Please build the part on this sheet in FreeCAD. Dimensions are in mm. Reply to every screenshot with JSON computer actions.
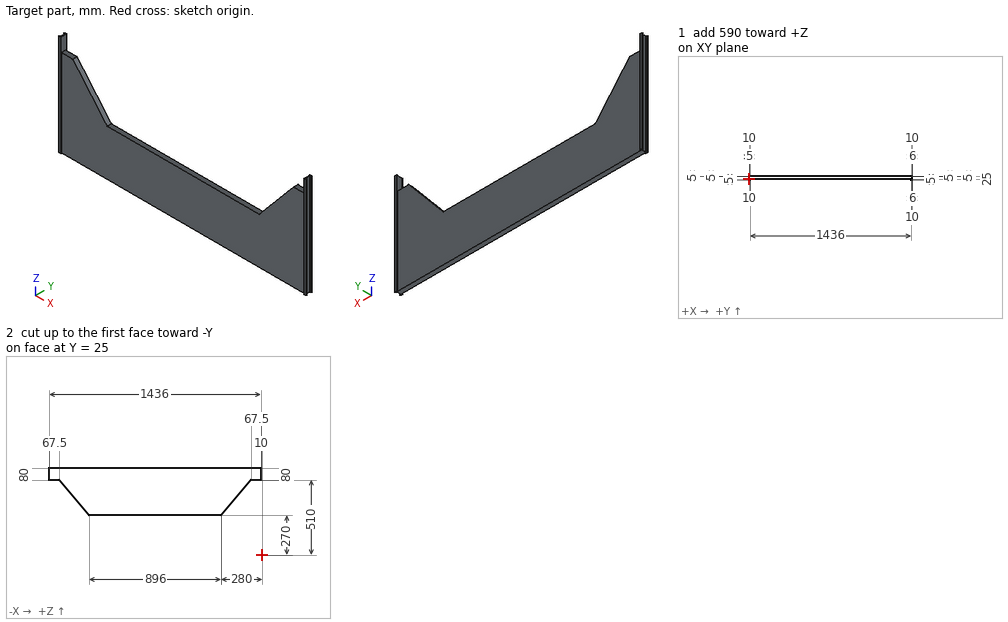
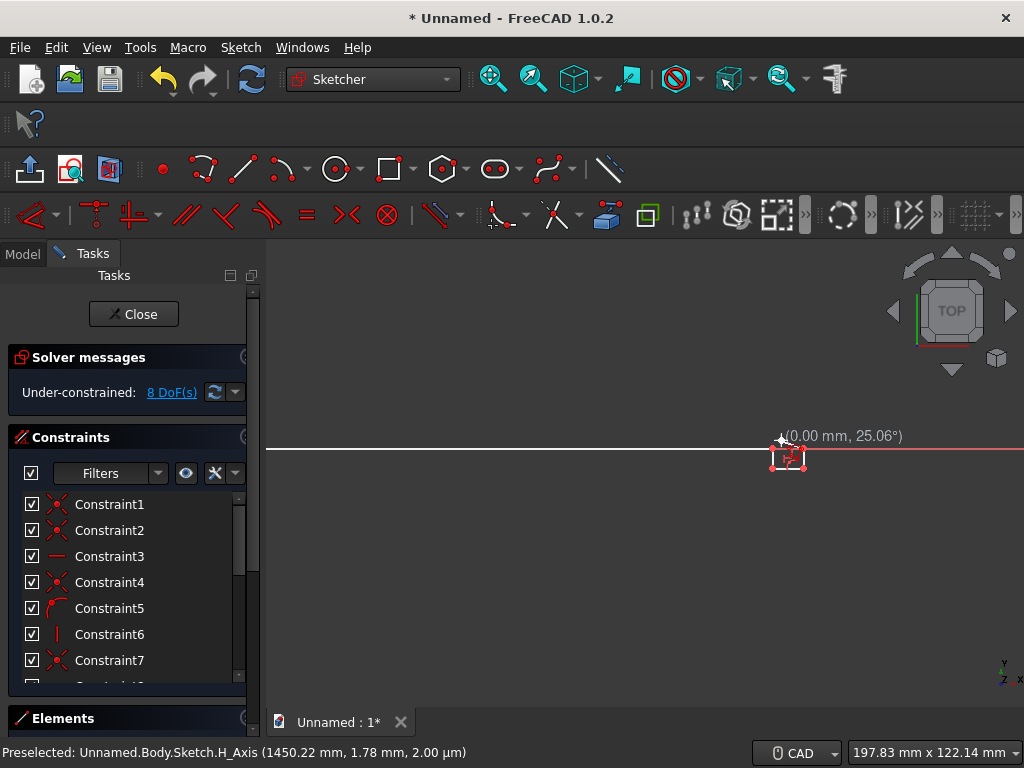
{"action": "scroll", "coordinate": [782, 479], "scroll_direction": "down", "scroll_amount": 13}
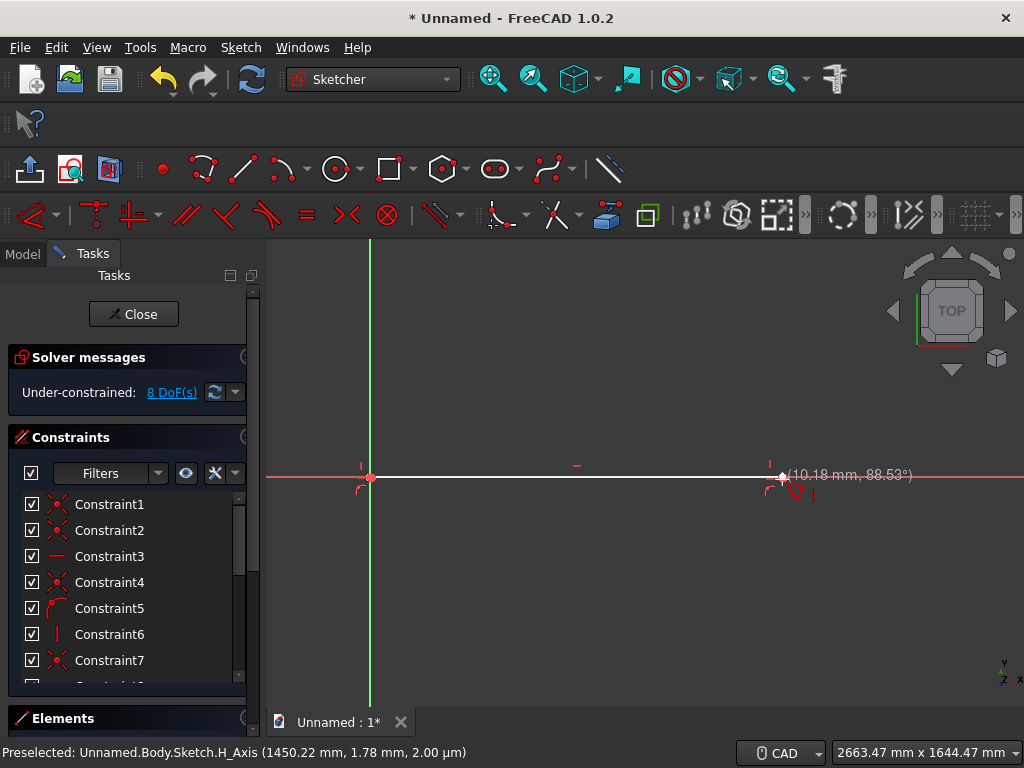
{"action": "scroll", "coordinate": [783, 470], "scroll_direction": "up", "scroll_amount": 5}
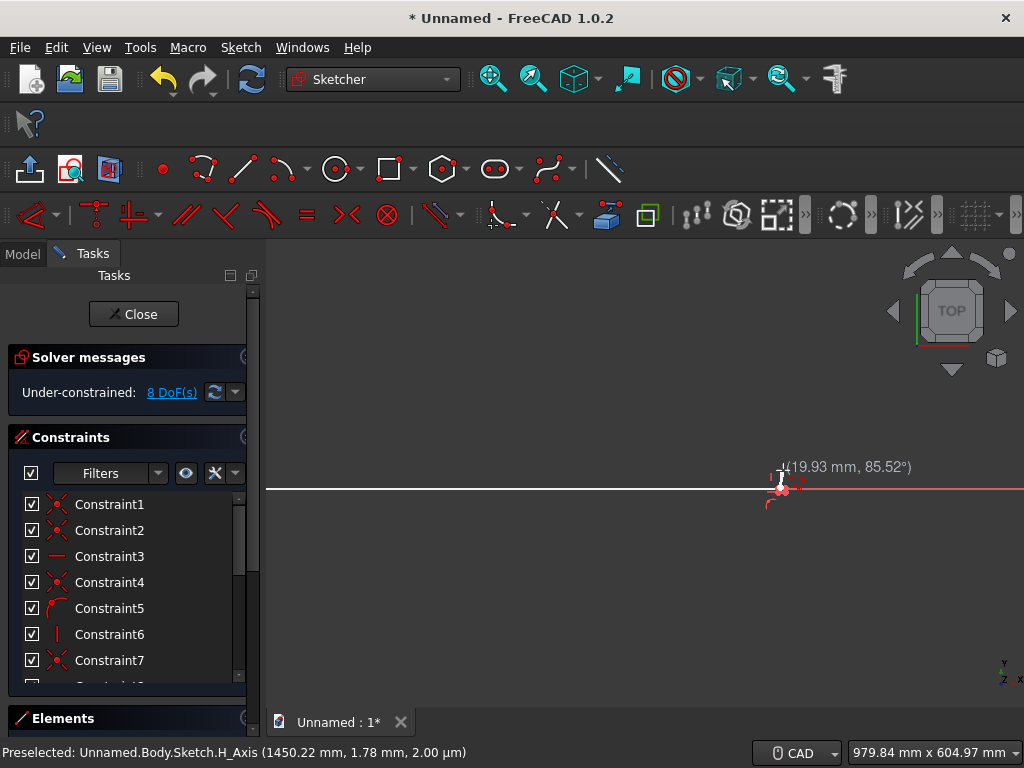
{"action": "left_click", "coordinate": [781, 469]}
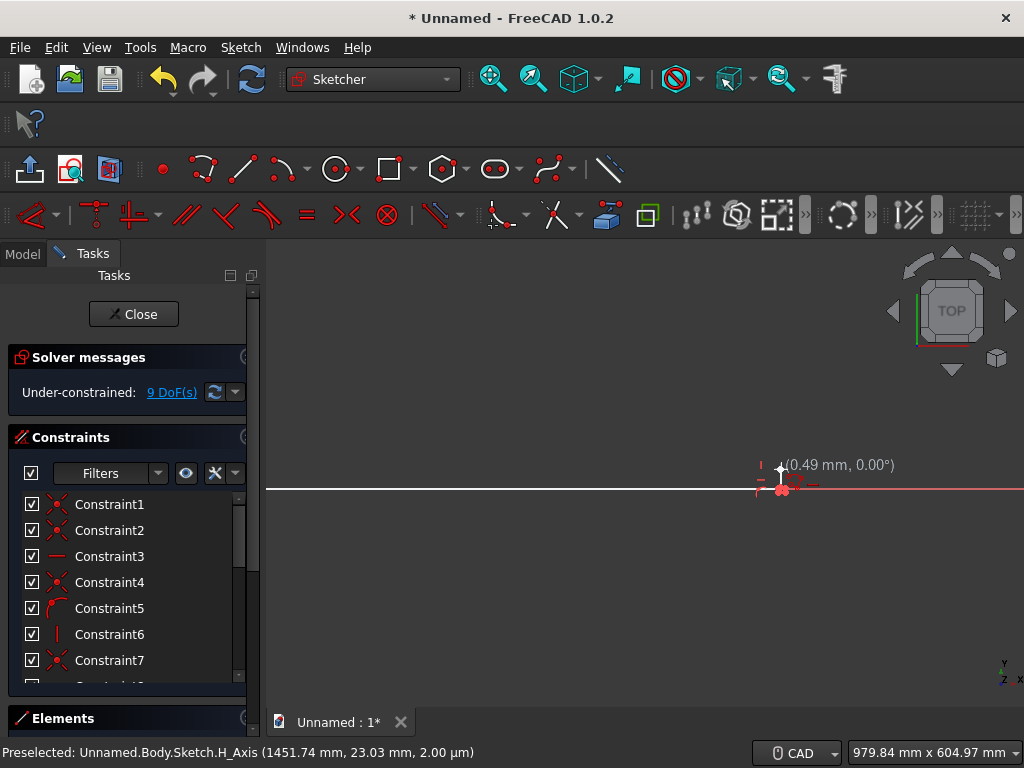
{"action": "scroll", "coordinate": [785, 469], "scroll_direction": "up", "scroll_amount": 7}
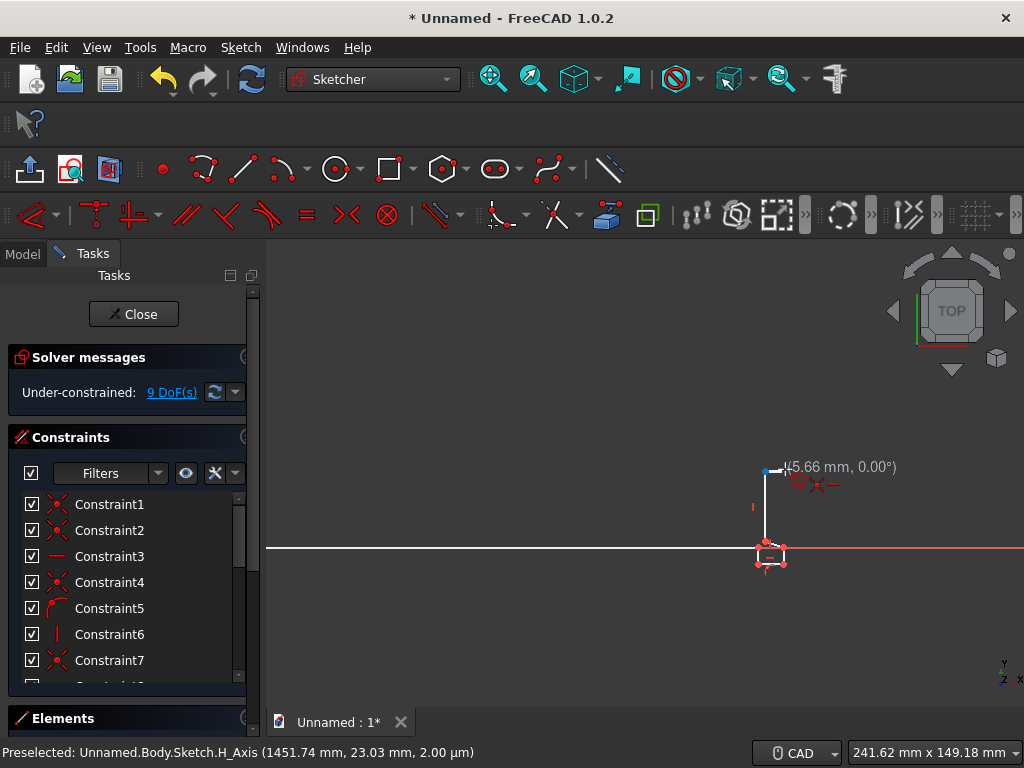
{"action": "left_click", "coordinate": [784, 467]}
{"action": "left_click", "coordinate": [784, 454]}
{"action": "left_click", "coordinate": [753, 454]}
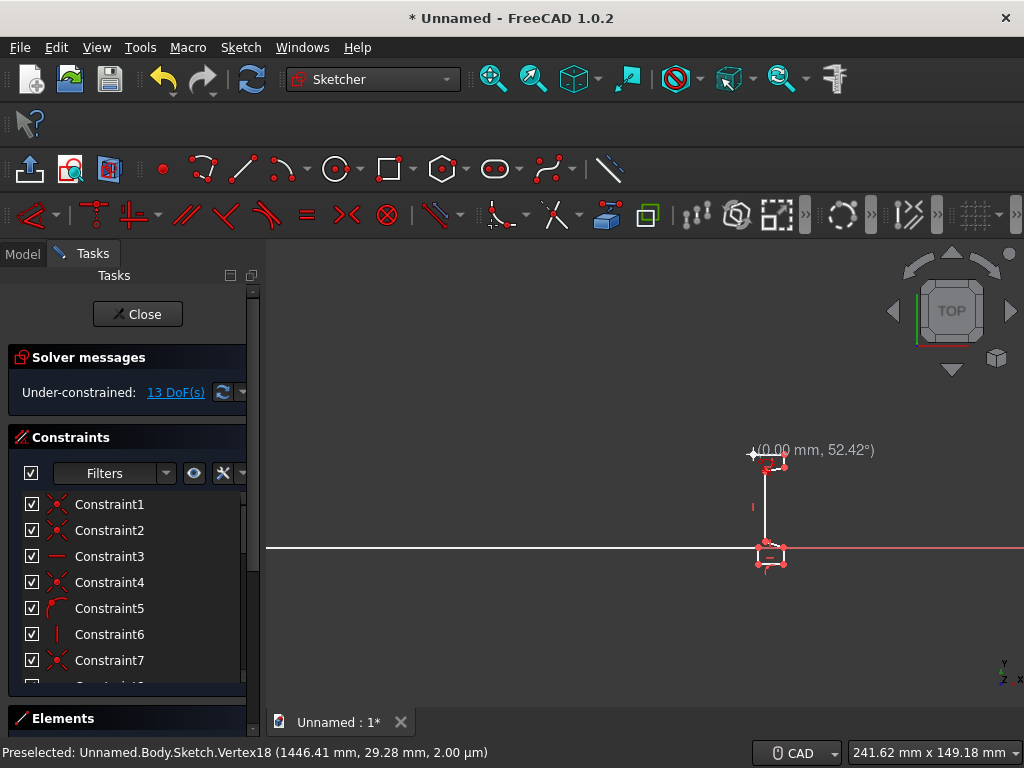
{"action": "scroll", "coordinate": [753, 469], "scroll_direction": "up", "scroll_amount": 2}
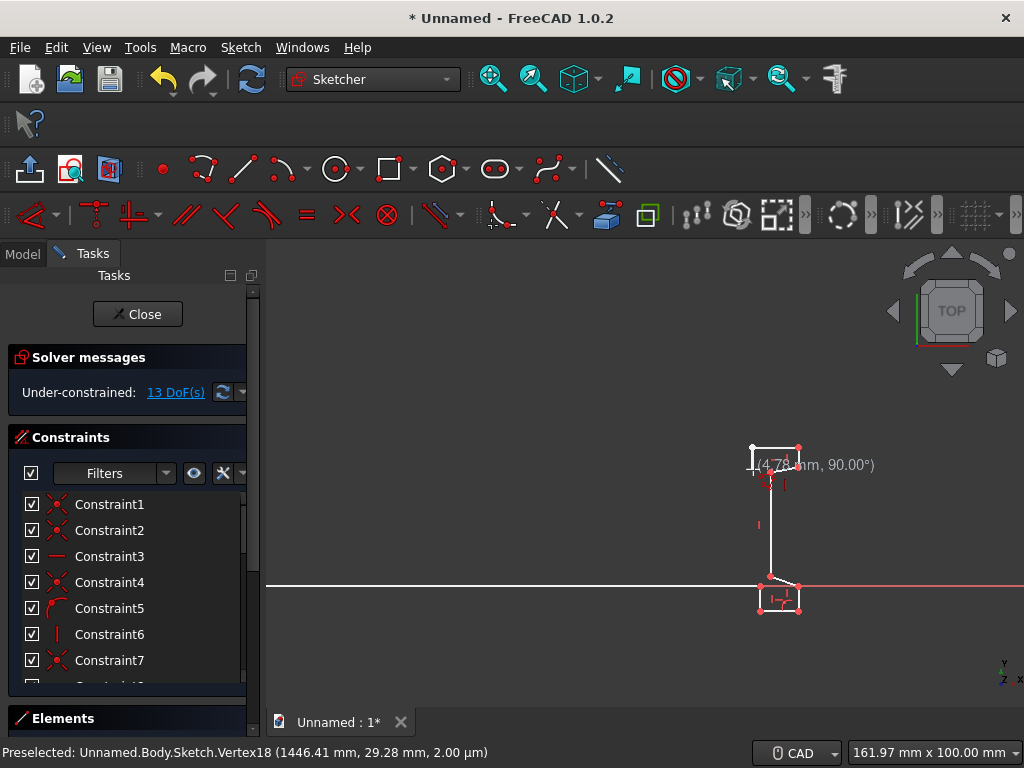
{"action": "left_click", "coordinate": [753, 469]}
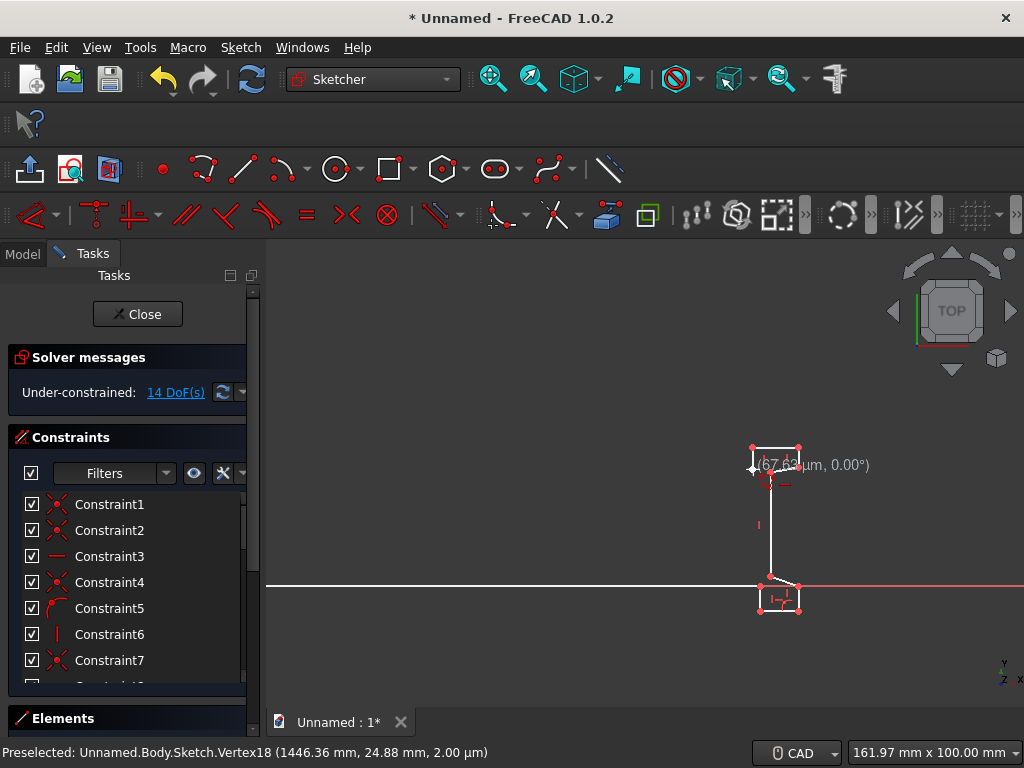
{"action": "scroll", "coordinate": [783, 469], "scroll_direction": "down", "scroll_amount": 14}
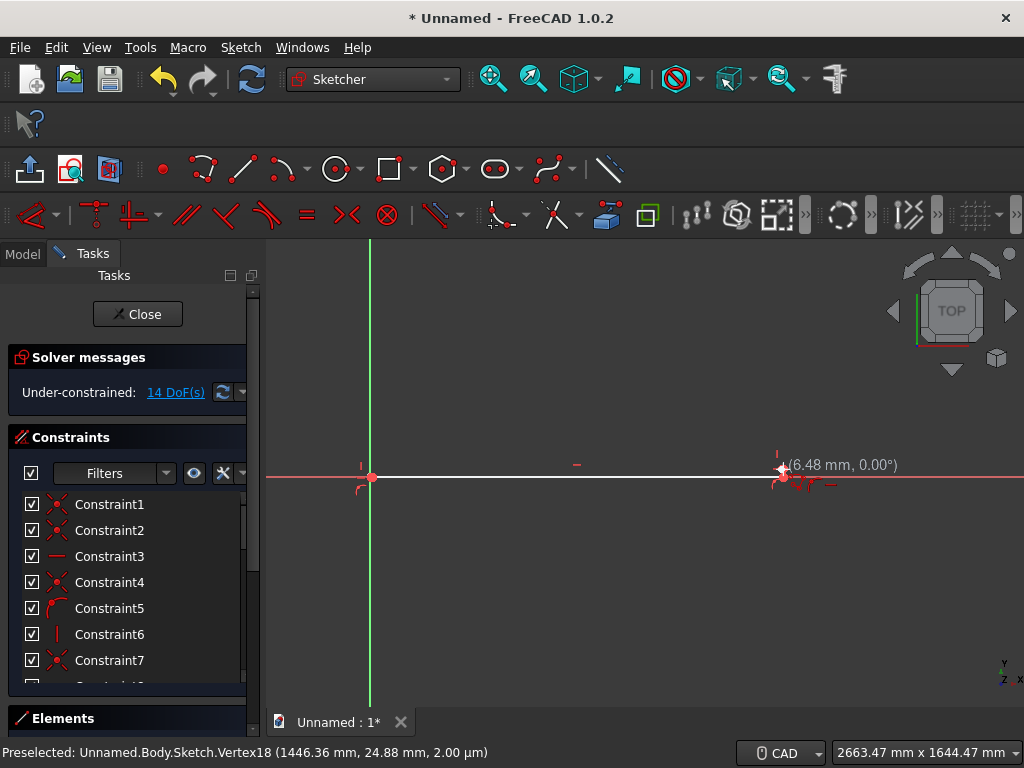
{"action": "scroll", "coordinate": [373, 469], "scroll_direction": "up", "scroll_amount": 9}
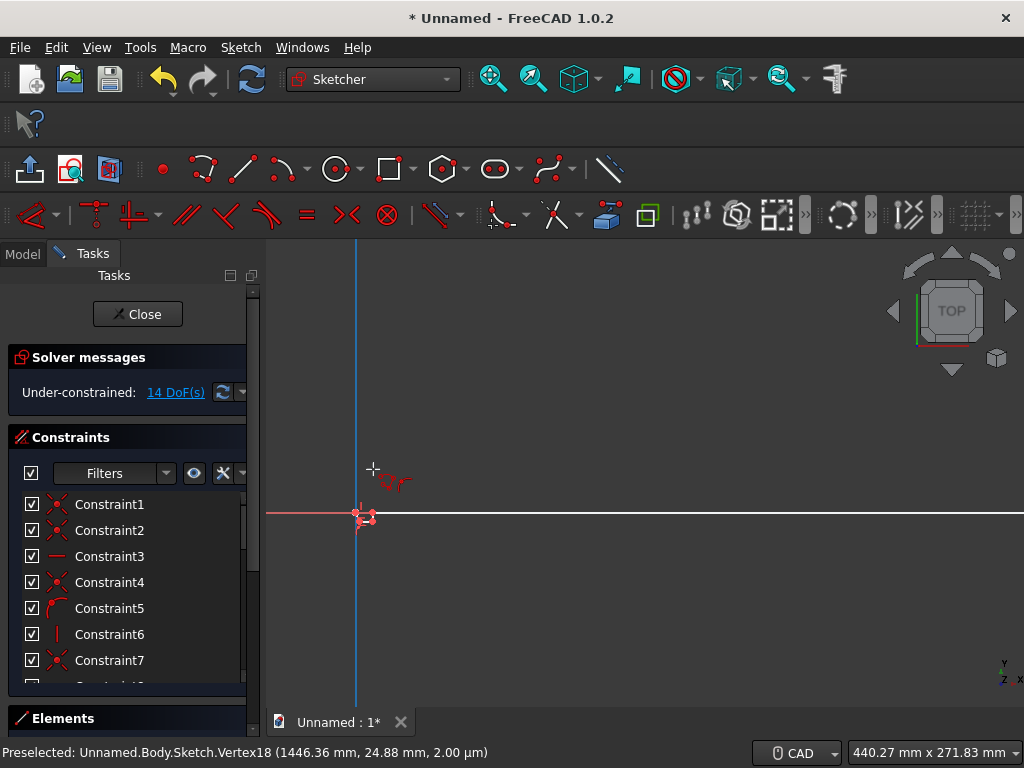
{"action": "left_click", "coordinate": [373, 469]}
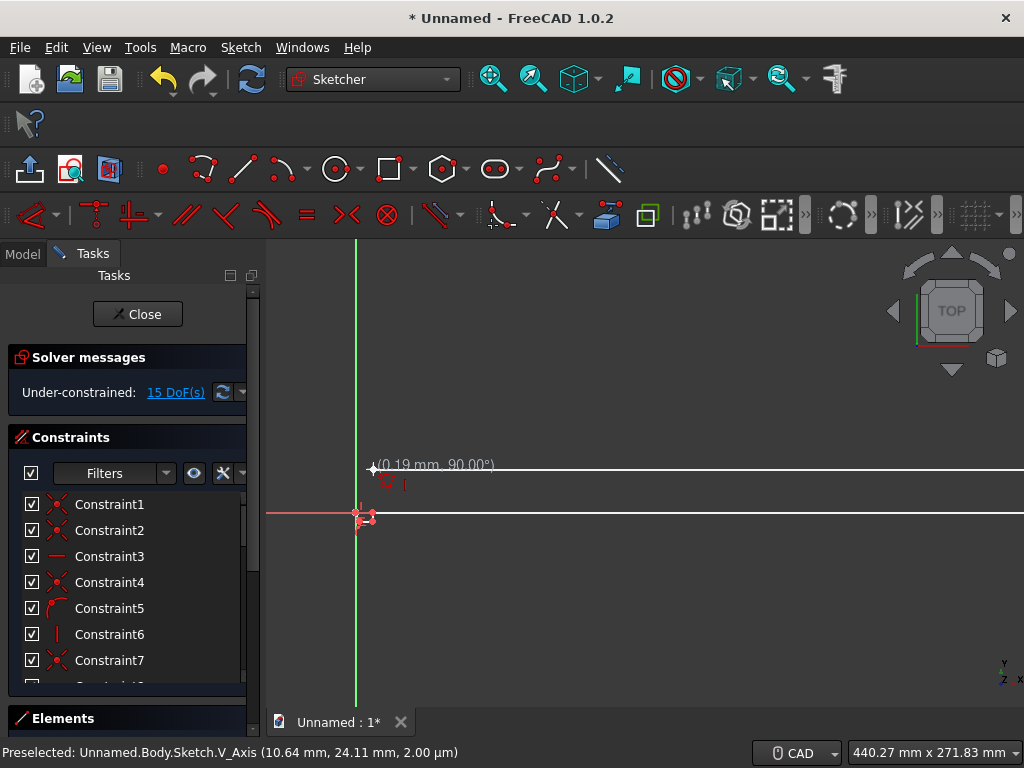
{"action": "scroll", "coordinate": [373, 461], "scroll_direction": "up", "scroll_amount": 4}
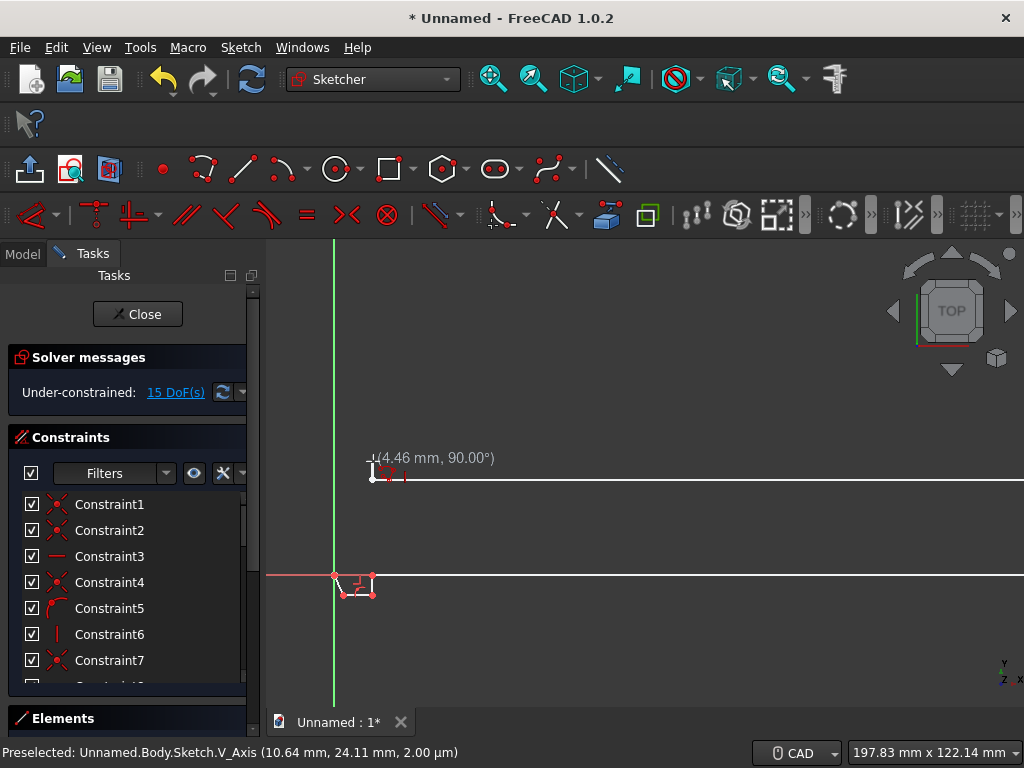
{"action": "left_click", "coordinate": [373, 460]}
{"action": "left_click", "coordinate": [334, 460]}
{"action": "left_click", "coordinate": [343, 479]}
{"action": "left_click", "coordinate": [353, 479]}
{"action": "left_click", "coordinate": [353, 566]}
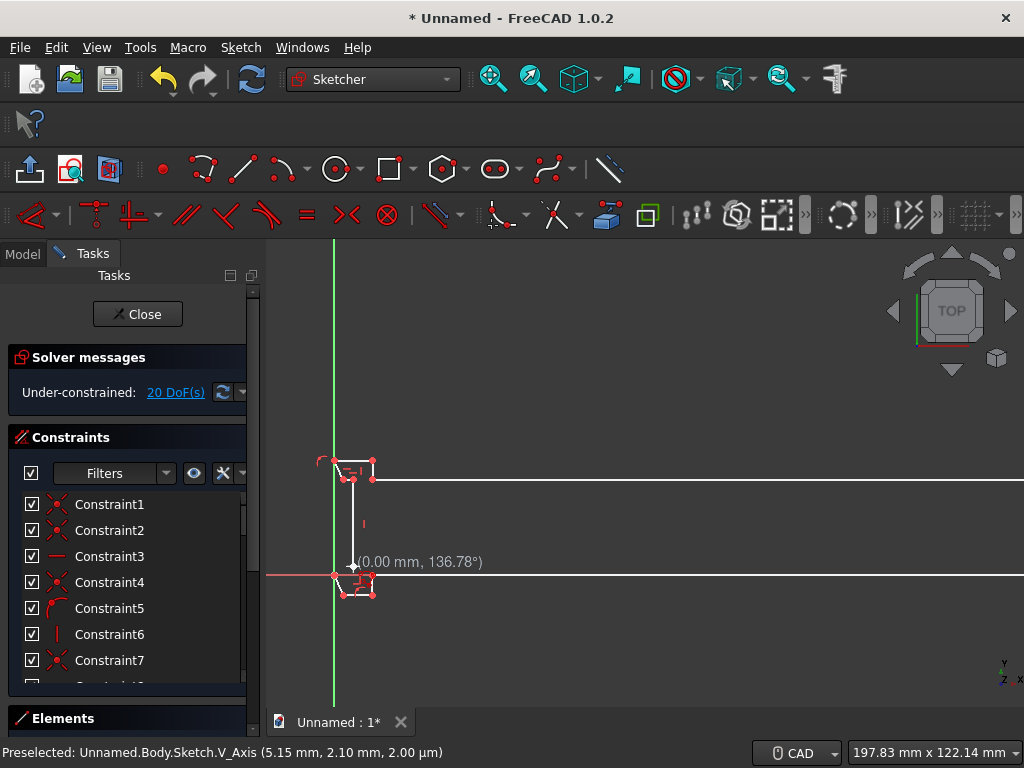
{"action": "scroll", "coordinate": [334, 575], "scroll_direction": "up", "scroll_amount": 3}